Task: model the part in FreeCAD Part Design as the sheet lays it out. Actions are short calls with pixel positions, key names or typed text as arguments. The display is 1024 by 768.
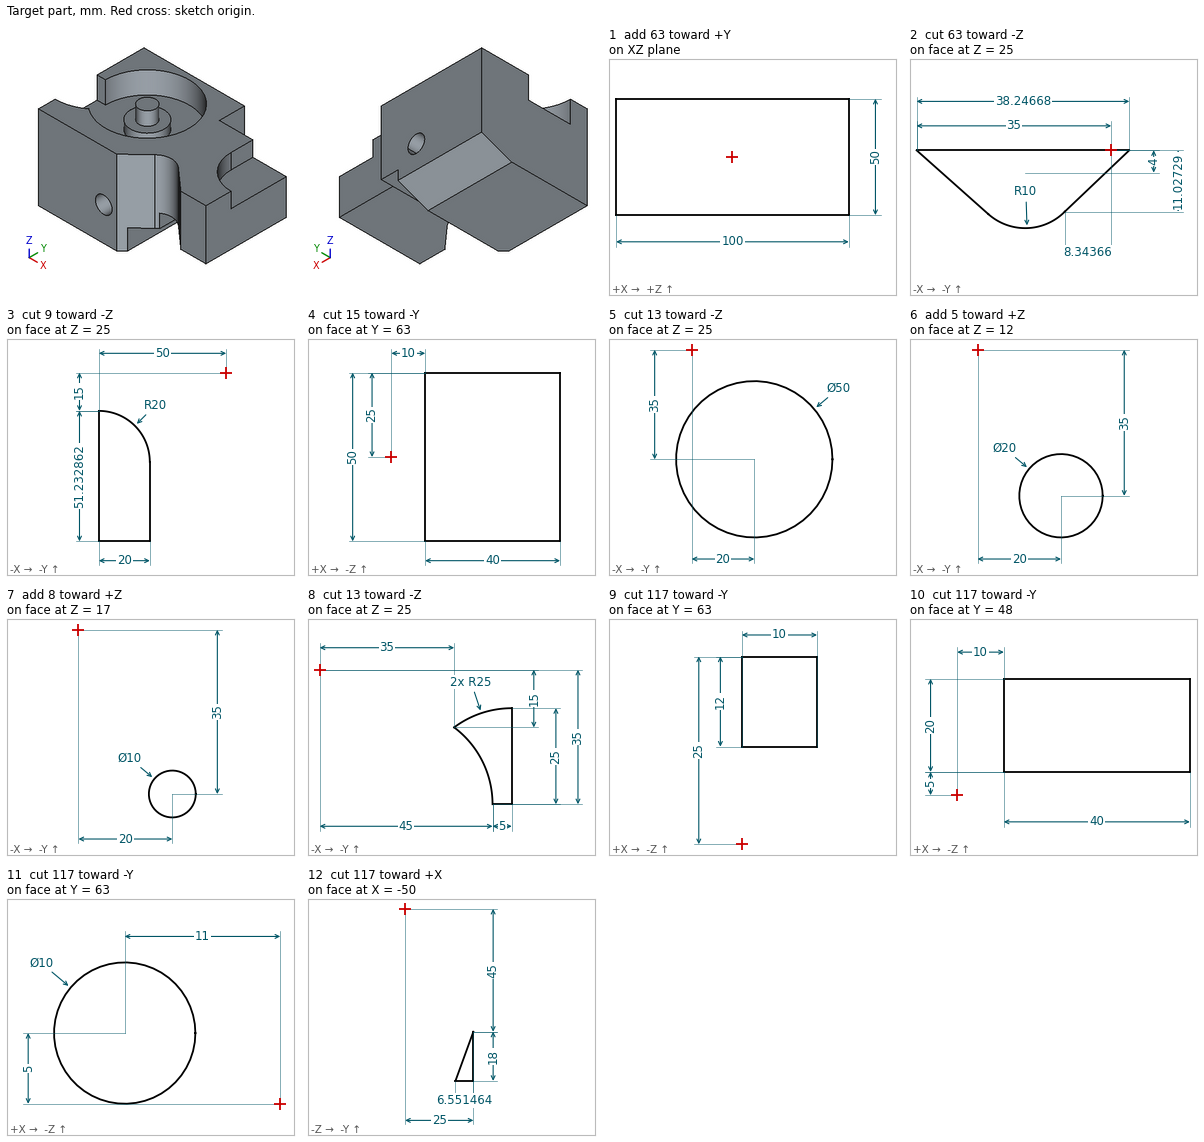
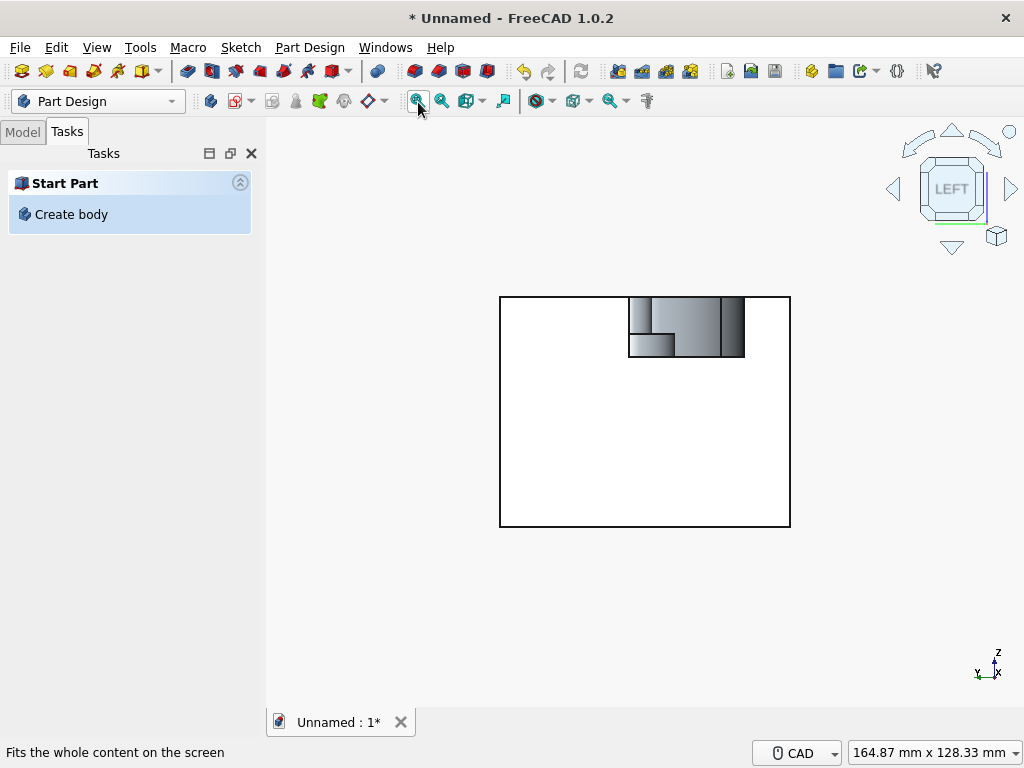
click(604, 444)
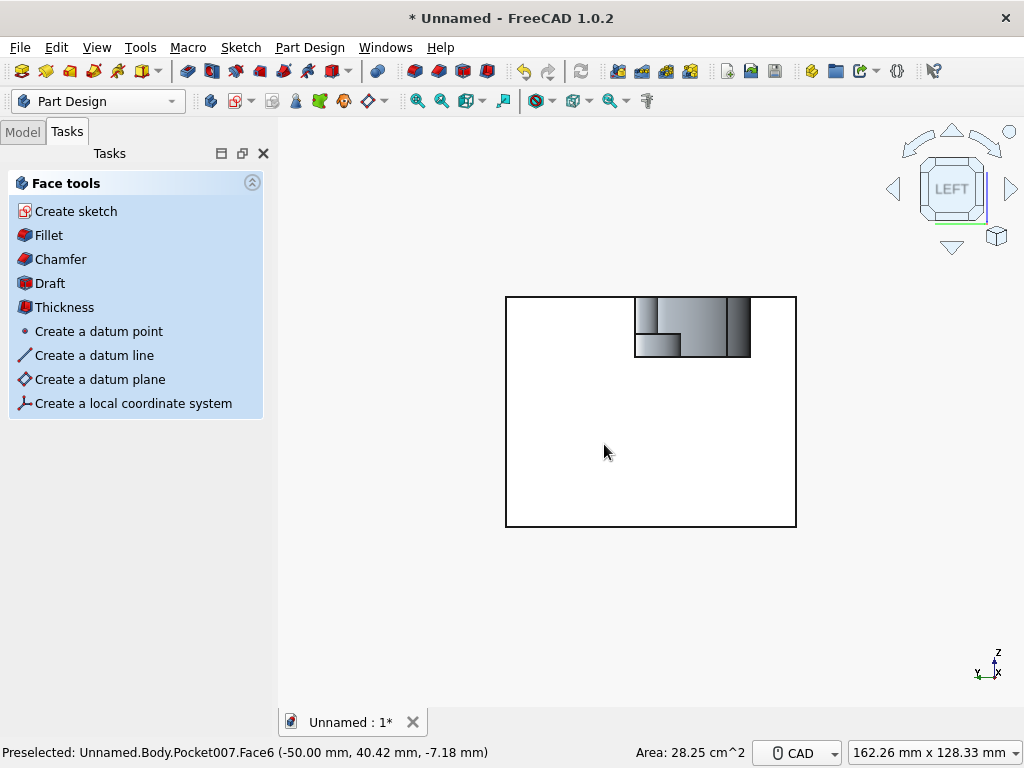
click(236, 102)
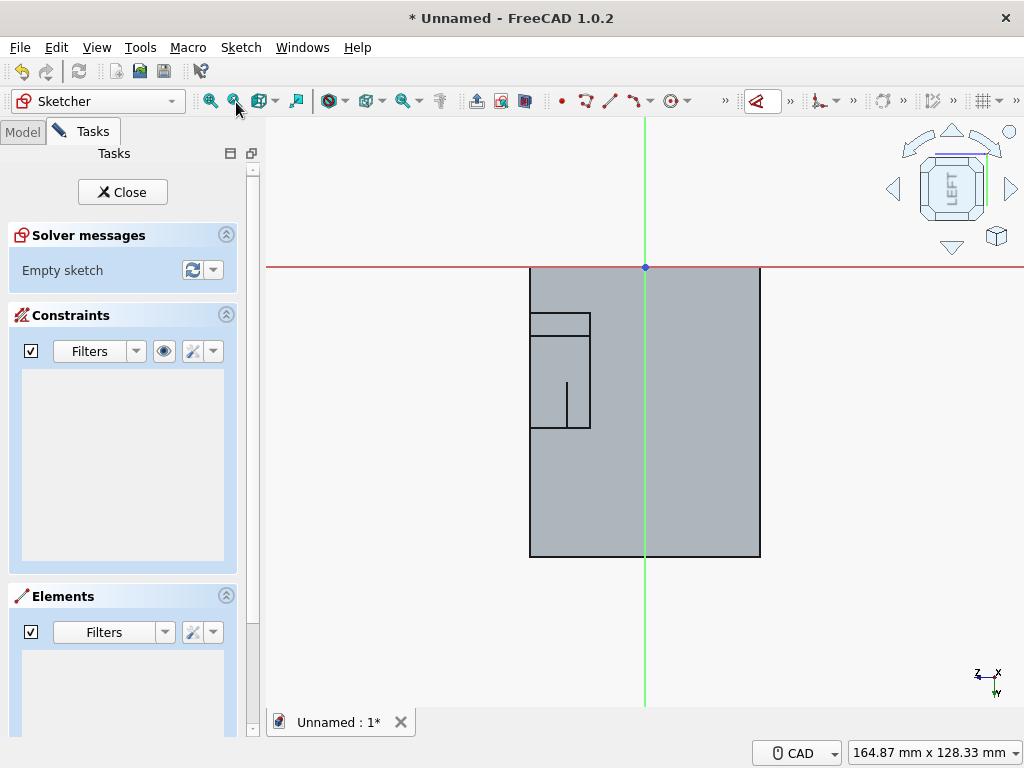
scroll(787, 542, up, 8)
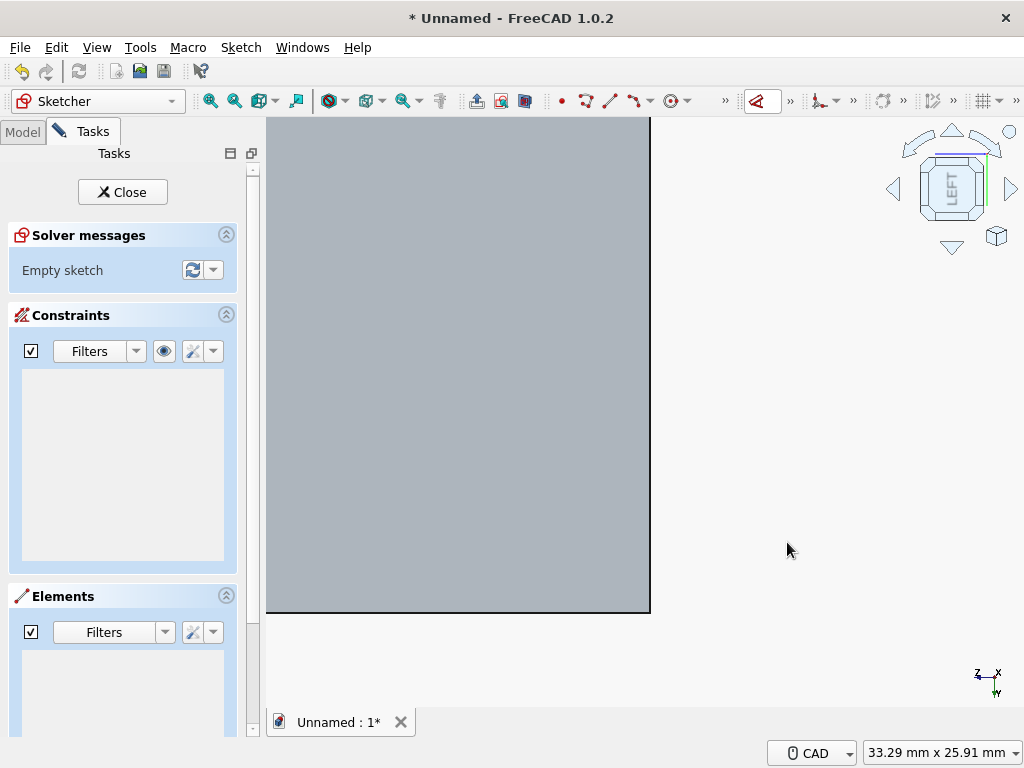
click(586, 102)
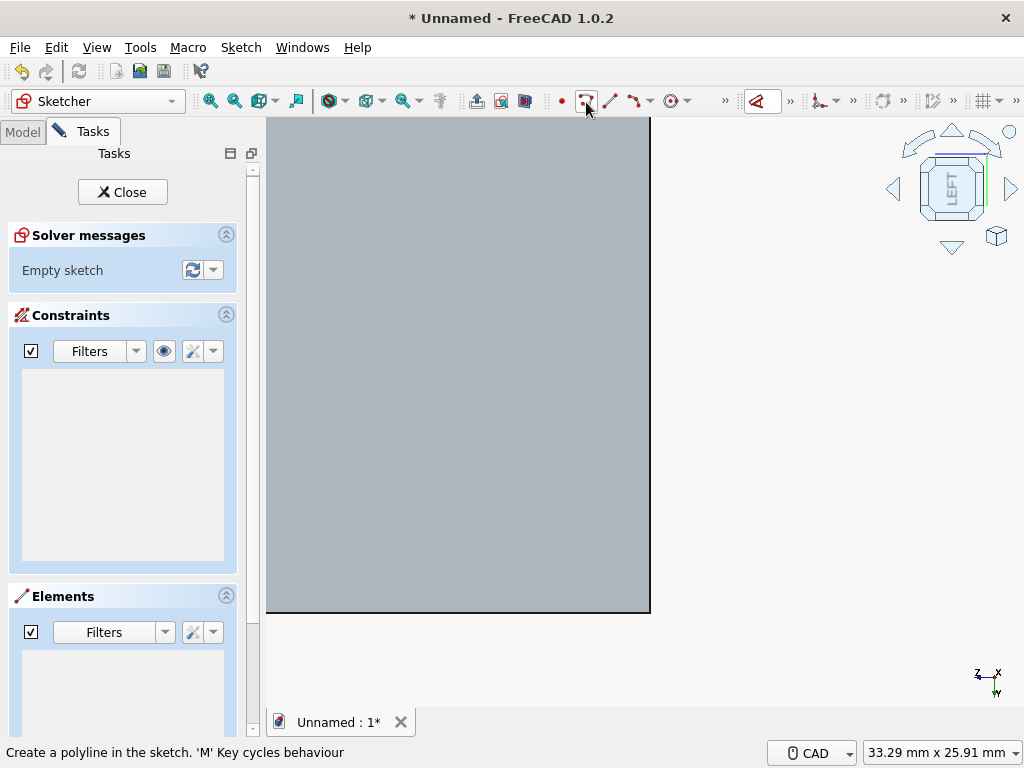
click(650, 203)
click(501, 613)
click(650, 613)
click(650, 204)
key(Escape)
key(Escape)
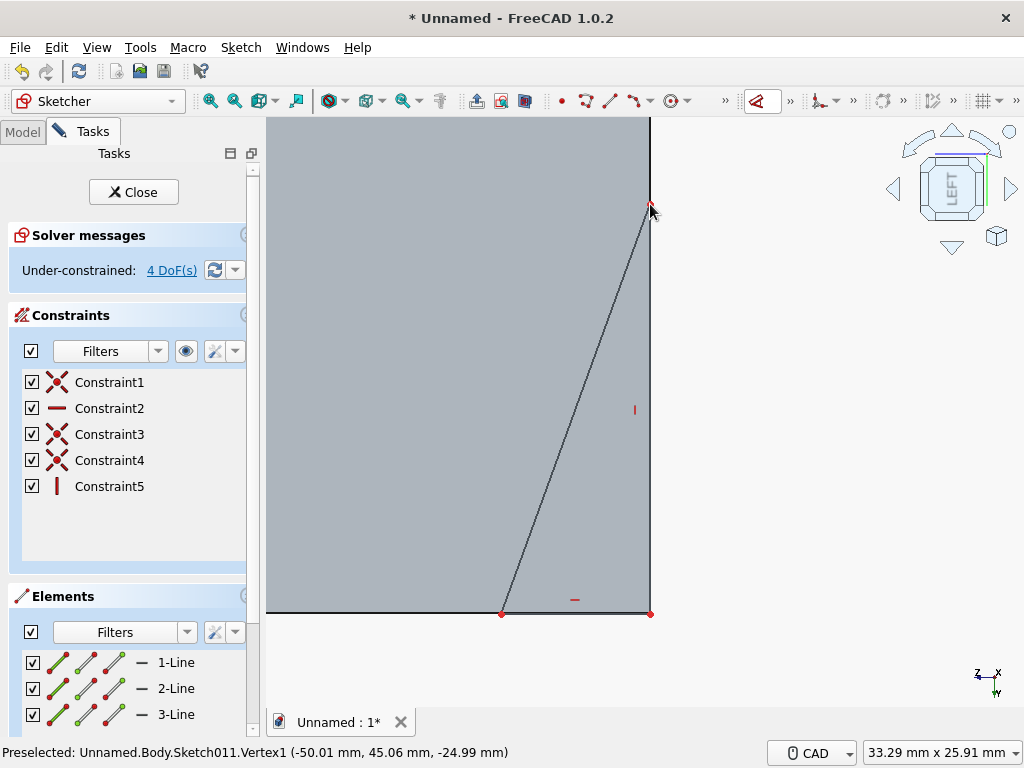
click(650, 491)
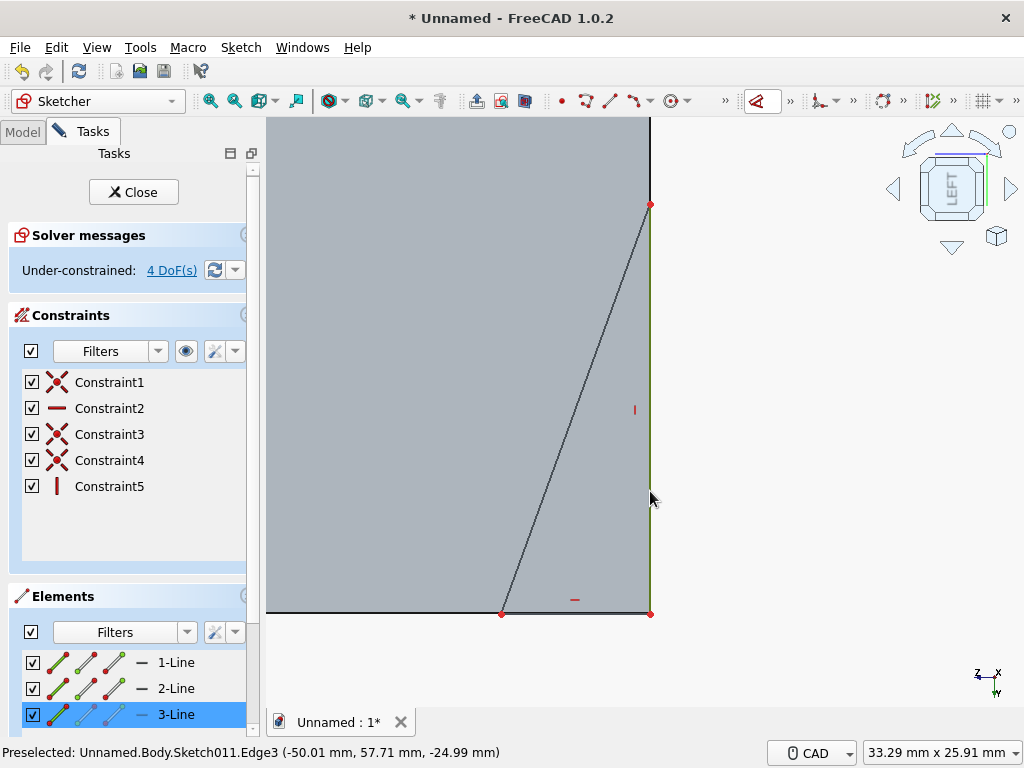
key(i)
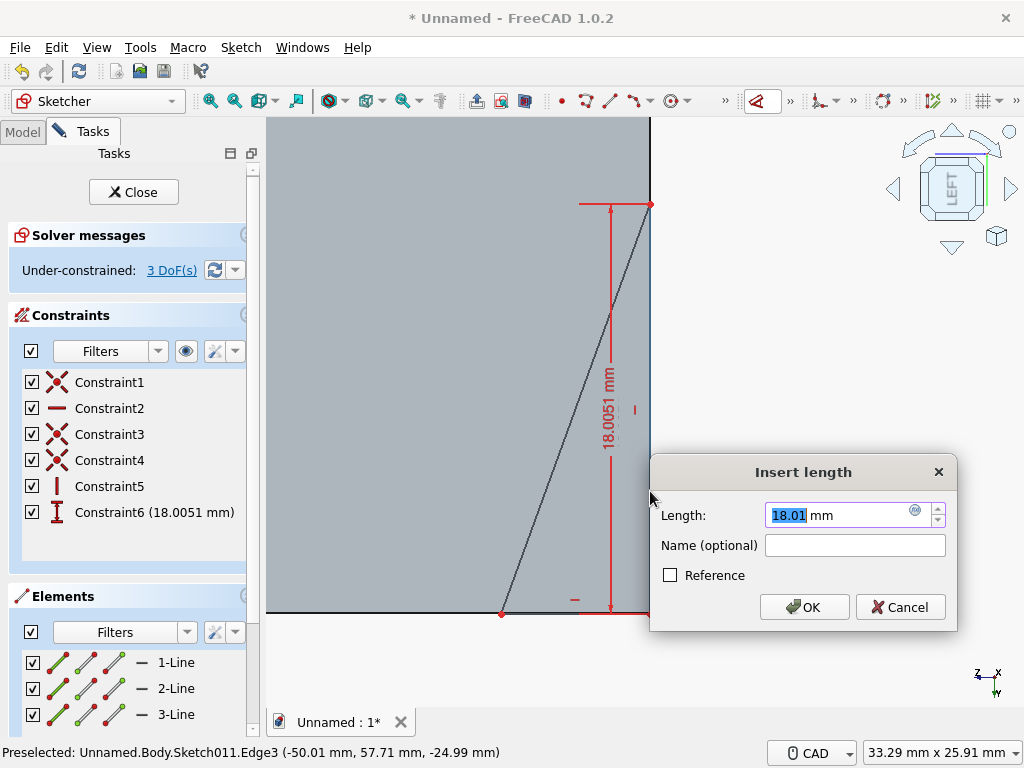
text(18)
key(Return)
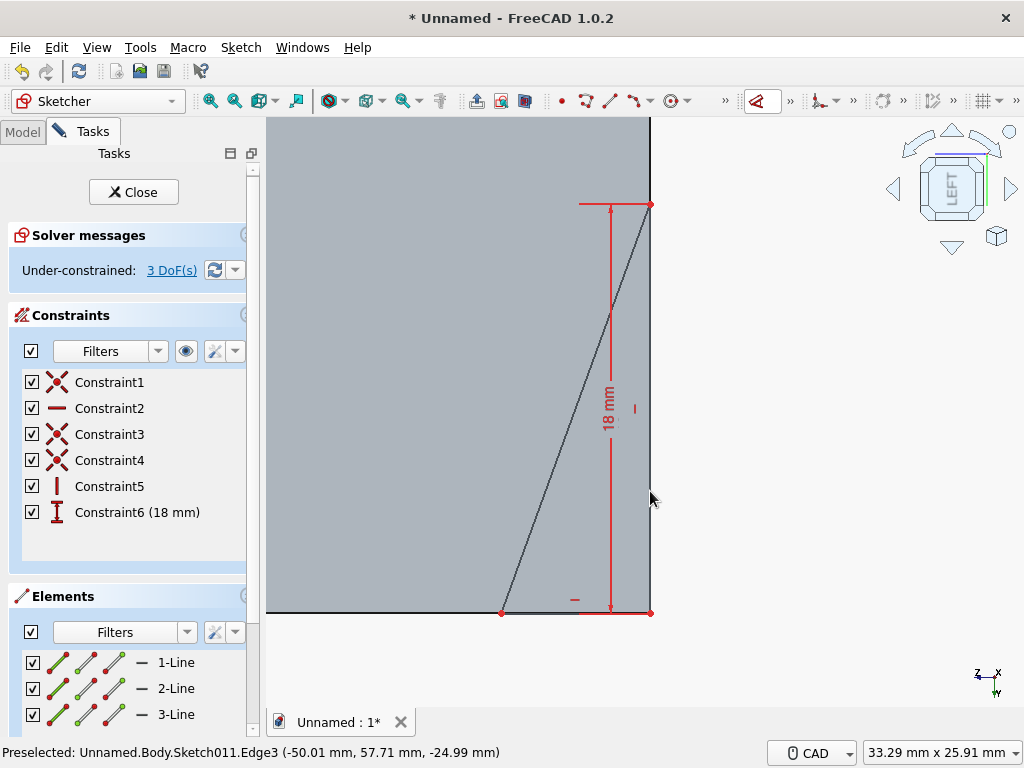
click(650, 204)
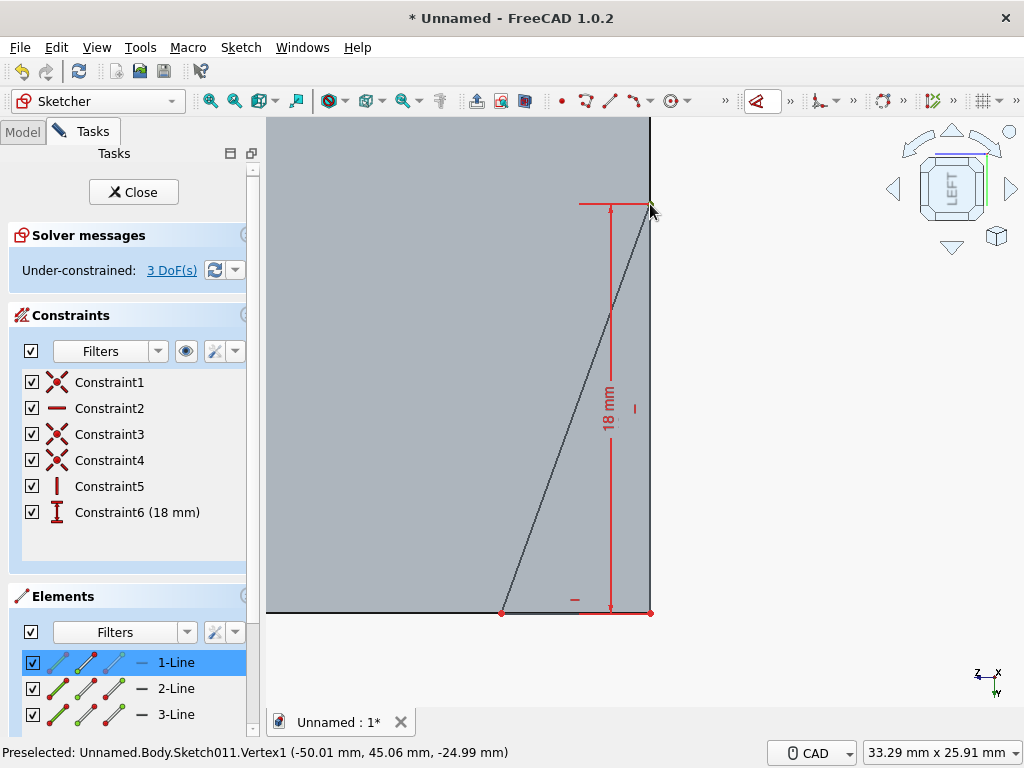
click(776, 102)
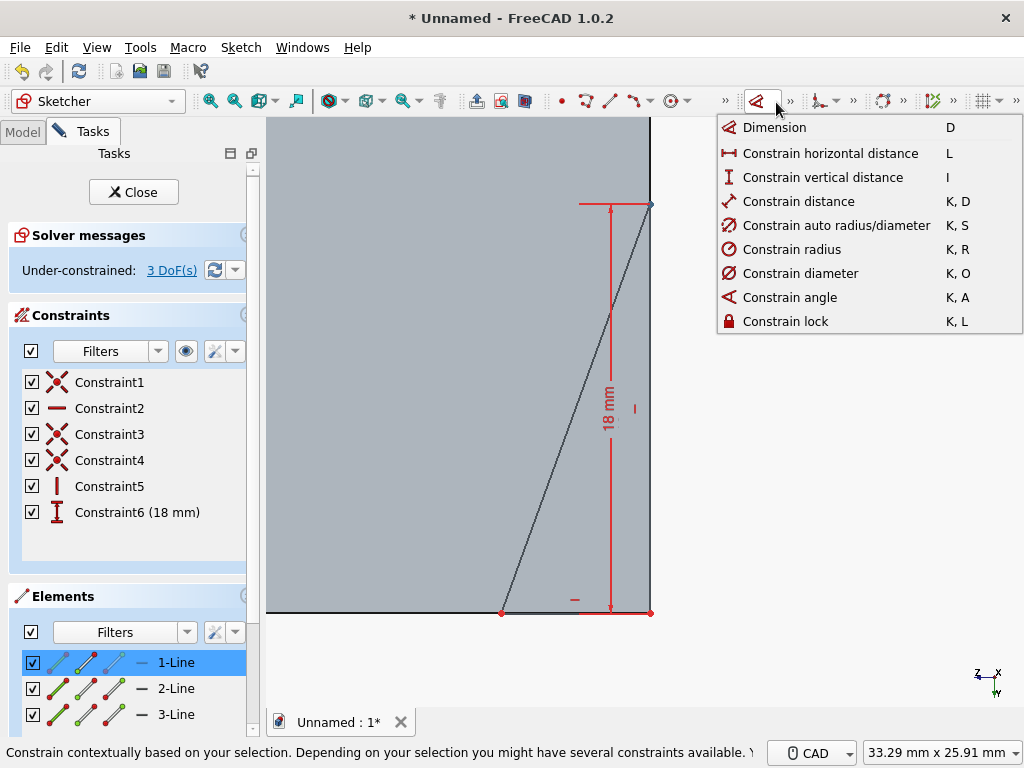
click(870, 153)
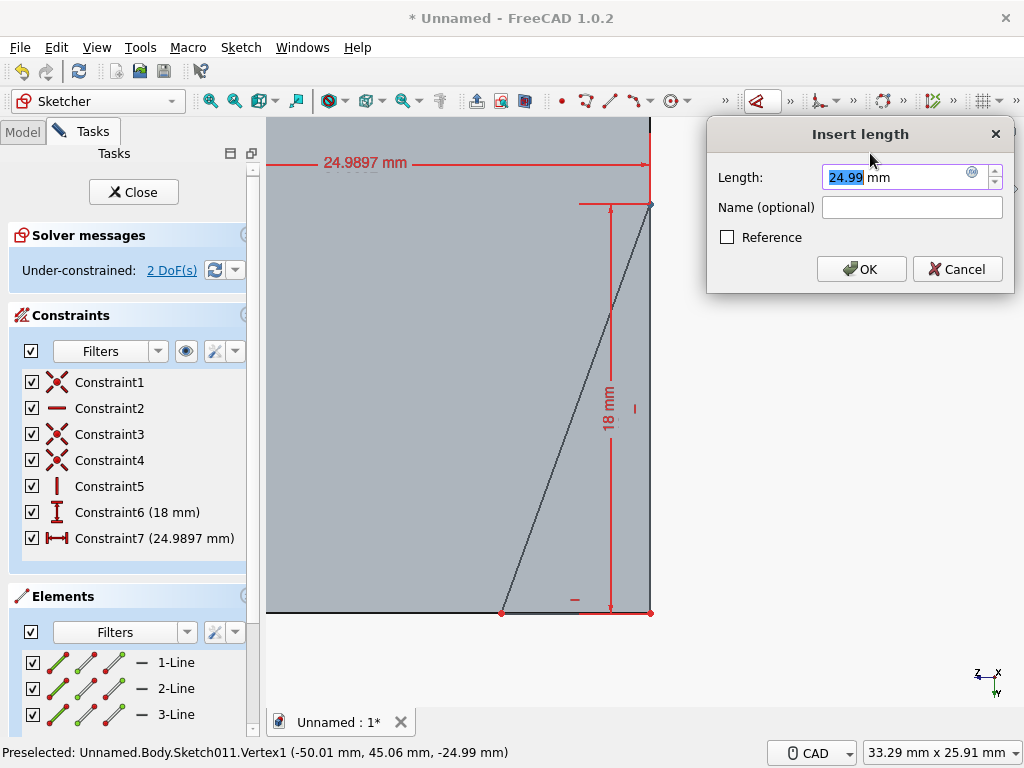
text(25)
key(Return)